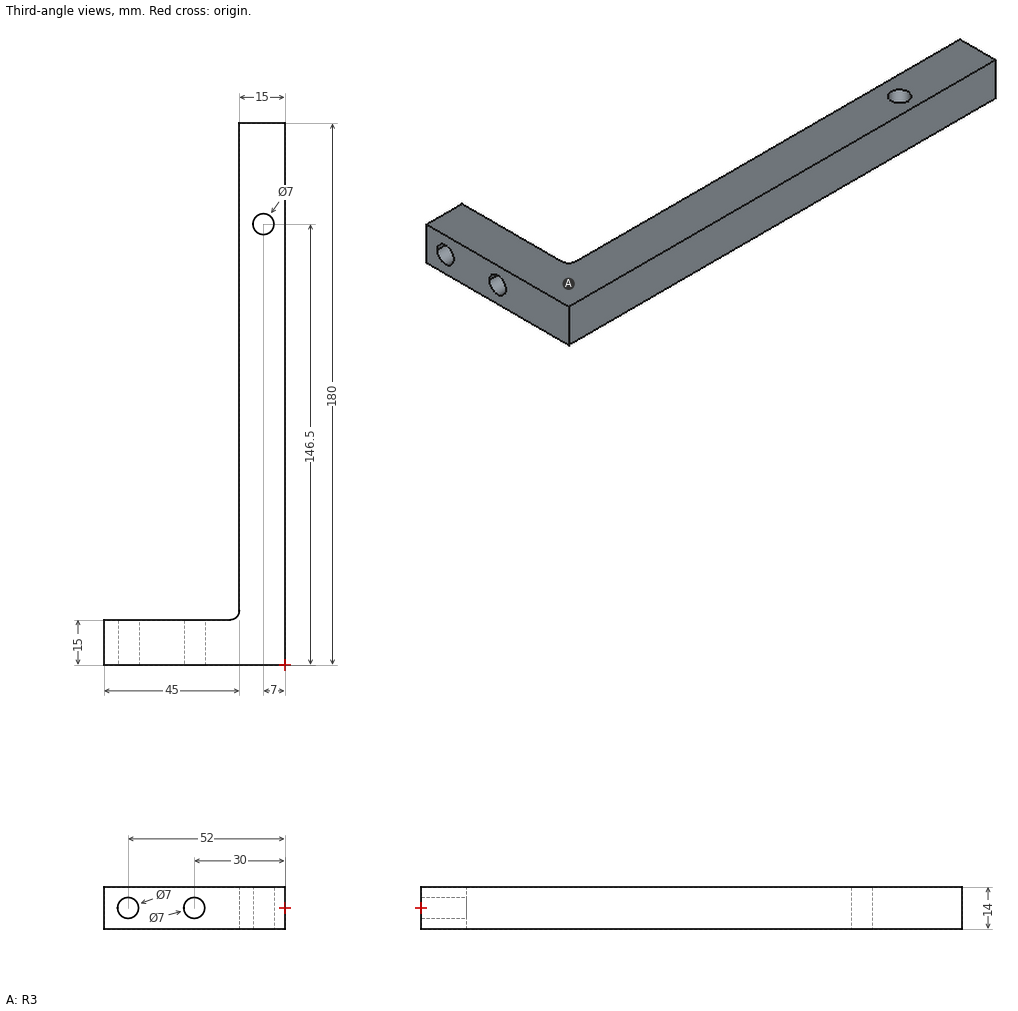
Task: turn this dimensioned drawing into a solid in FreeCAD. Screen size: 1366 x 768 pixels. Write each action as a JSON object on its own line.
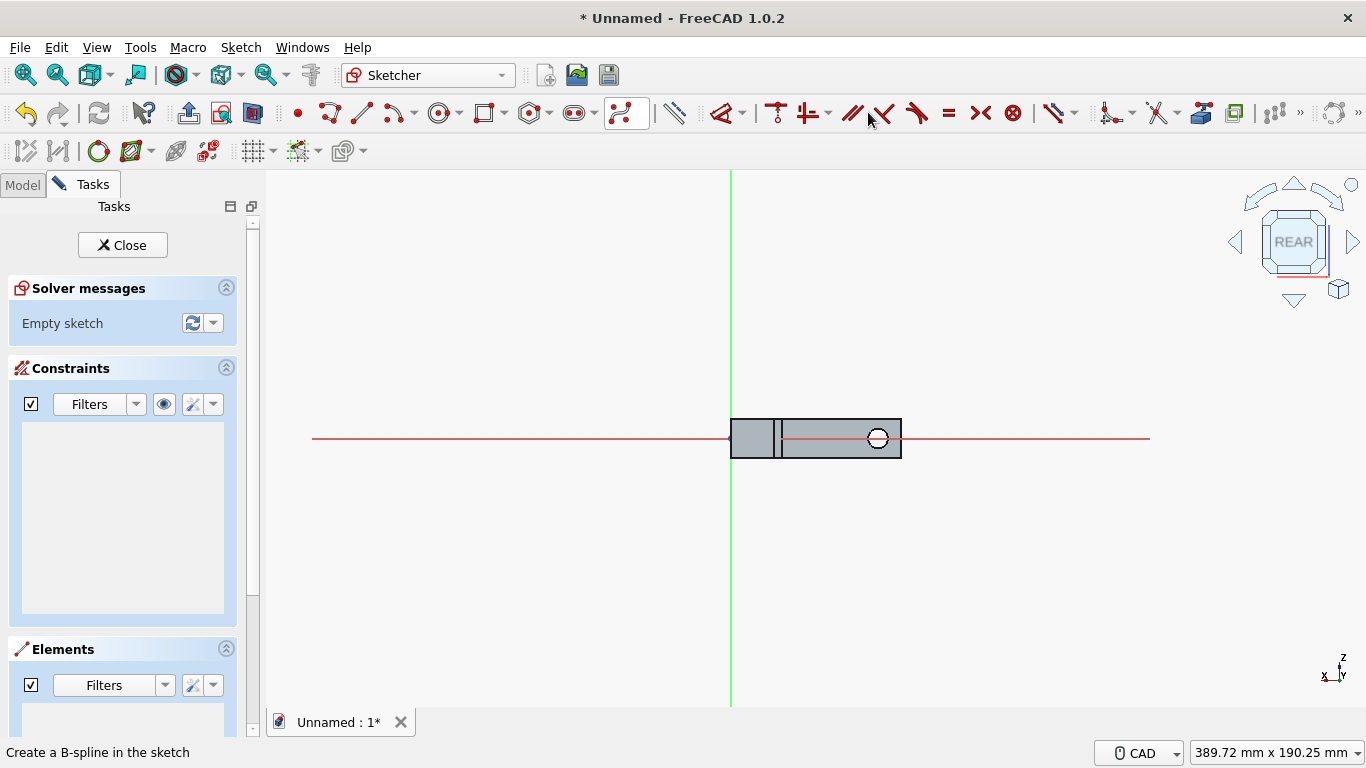
{"action": "left_click", "coordinate": [254, 114]}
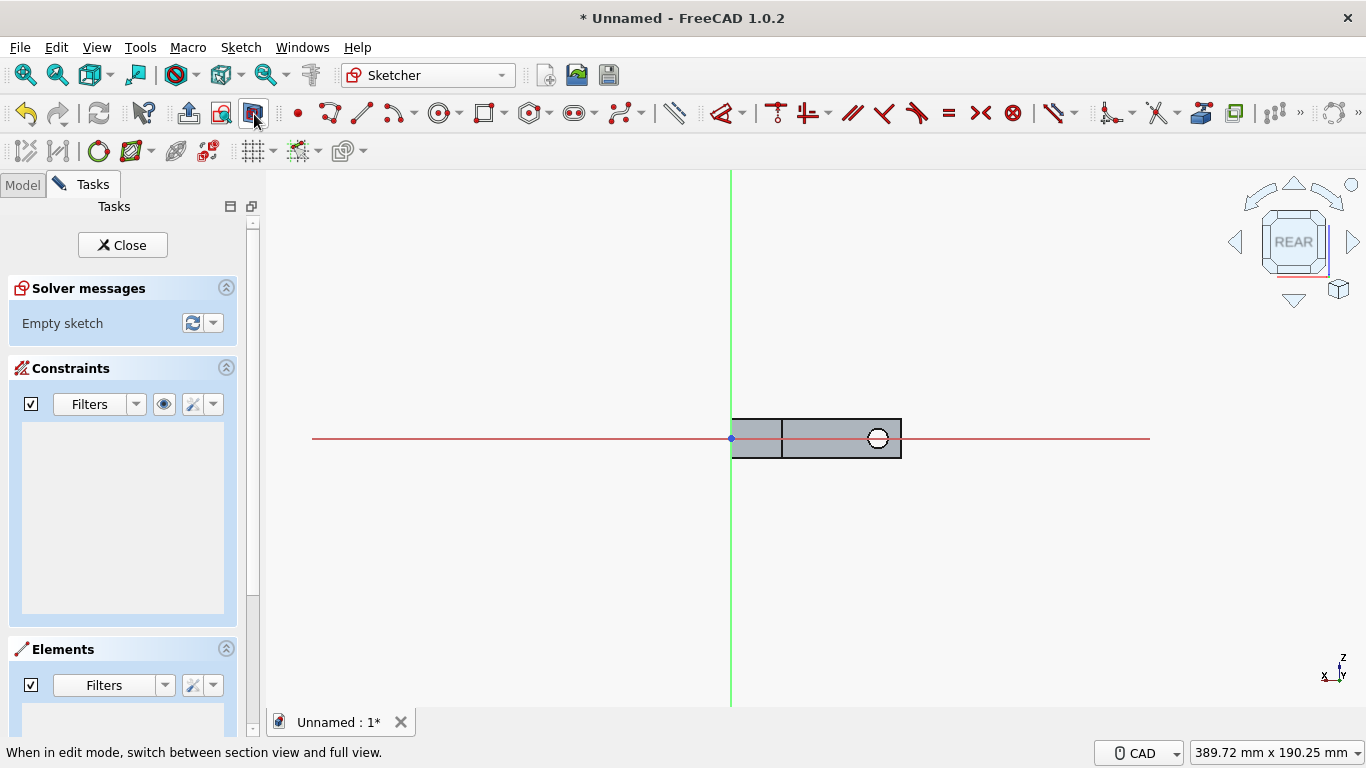
{"action": "scroll", "coordinate": [820, 439], "scroll_direction": "up", "scroll_amount": 14}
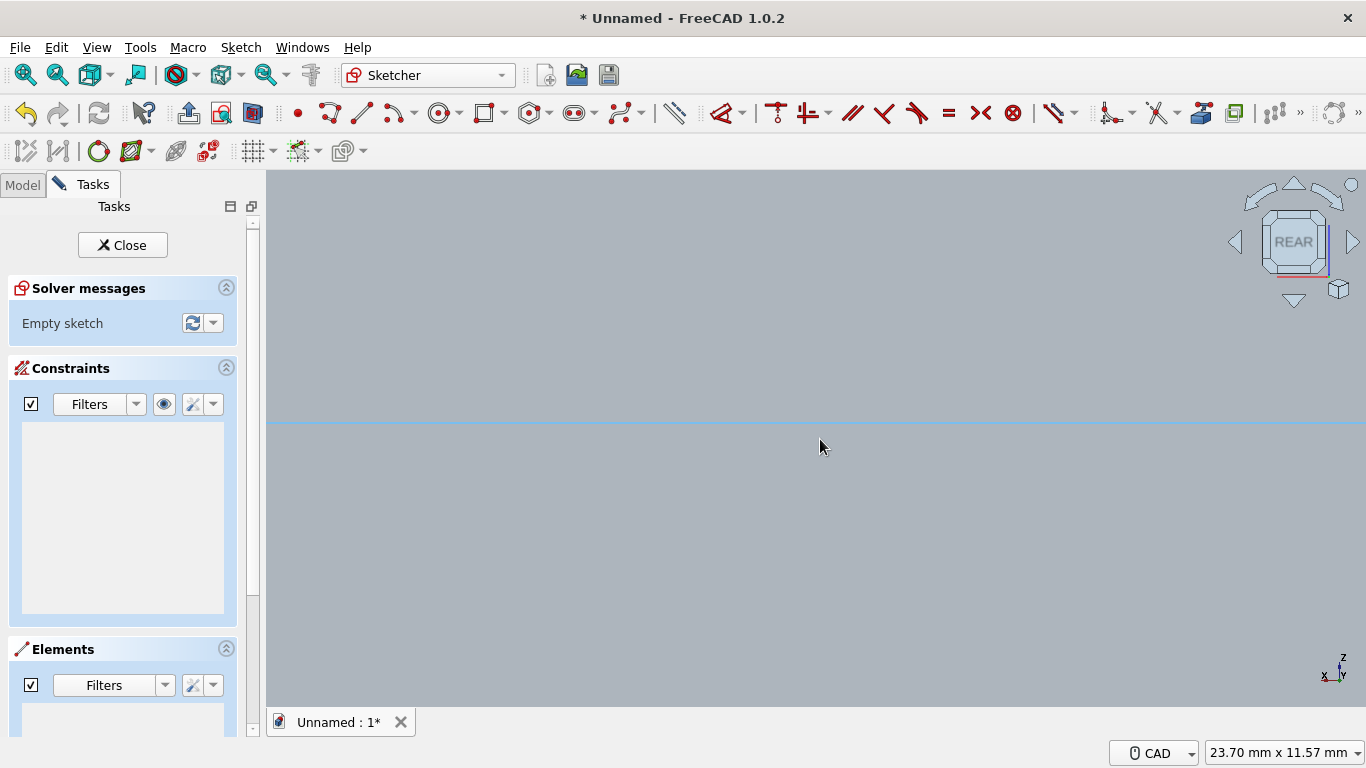
{"action": "left_click", "coordinate": [440, 114]}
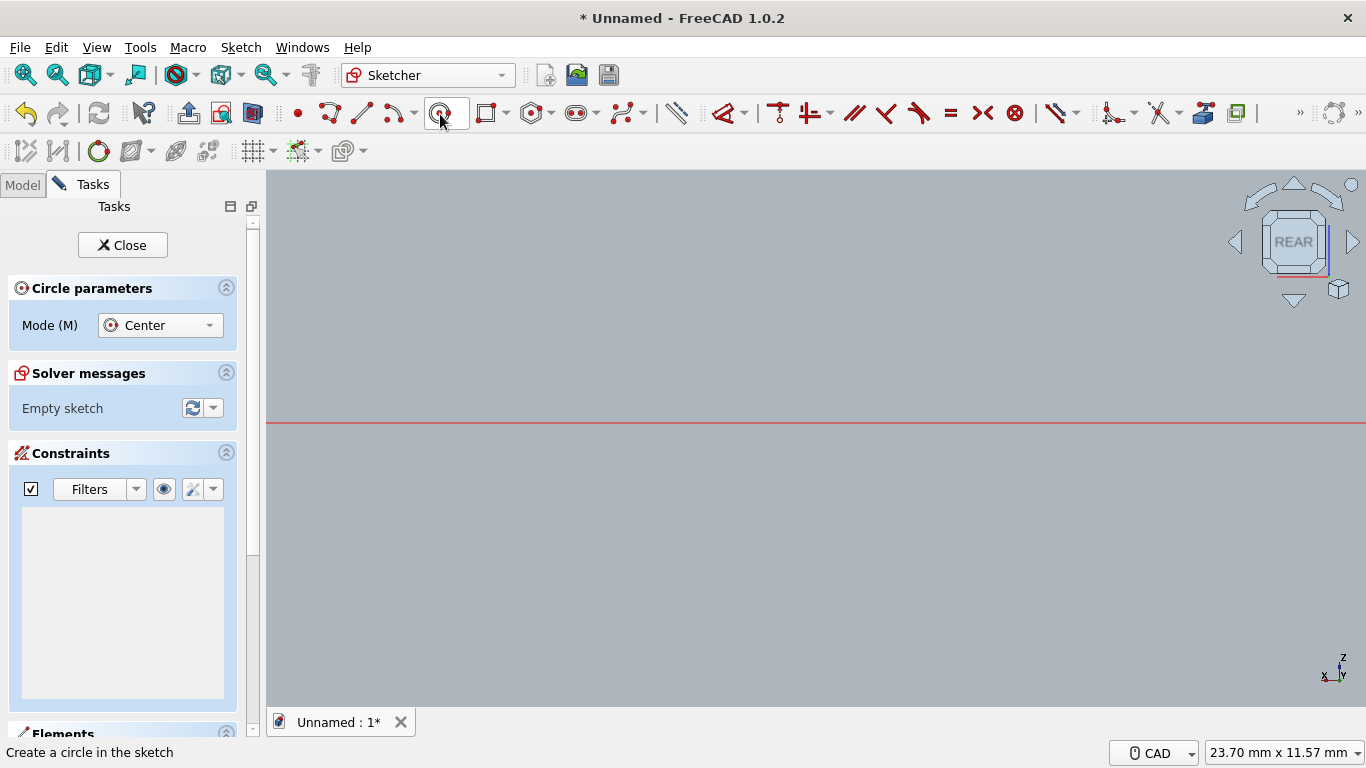
{"action": "left_click", "coordinate": [746, 423]}
{"action": "mouse_move", "coordinate": [861, 308]}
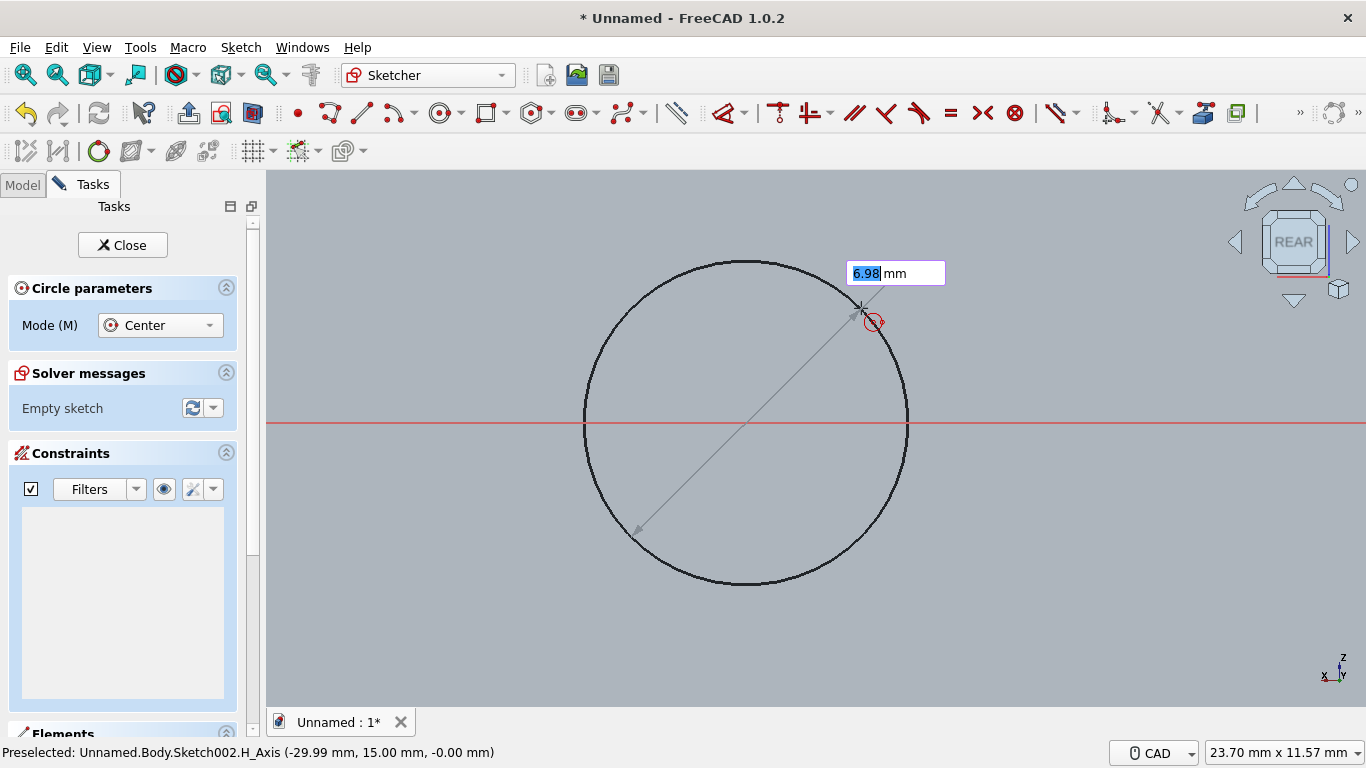
{"action": "type", "text": "7"}
{"action": "key", "text": "Return"}
{"action": "key", "text": "Escape"}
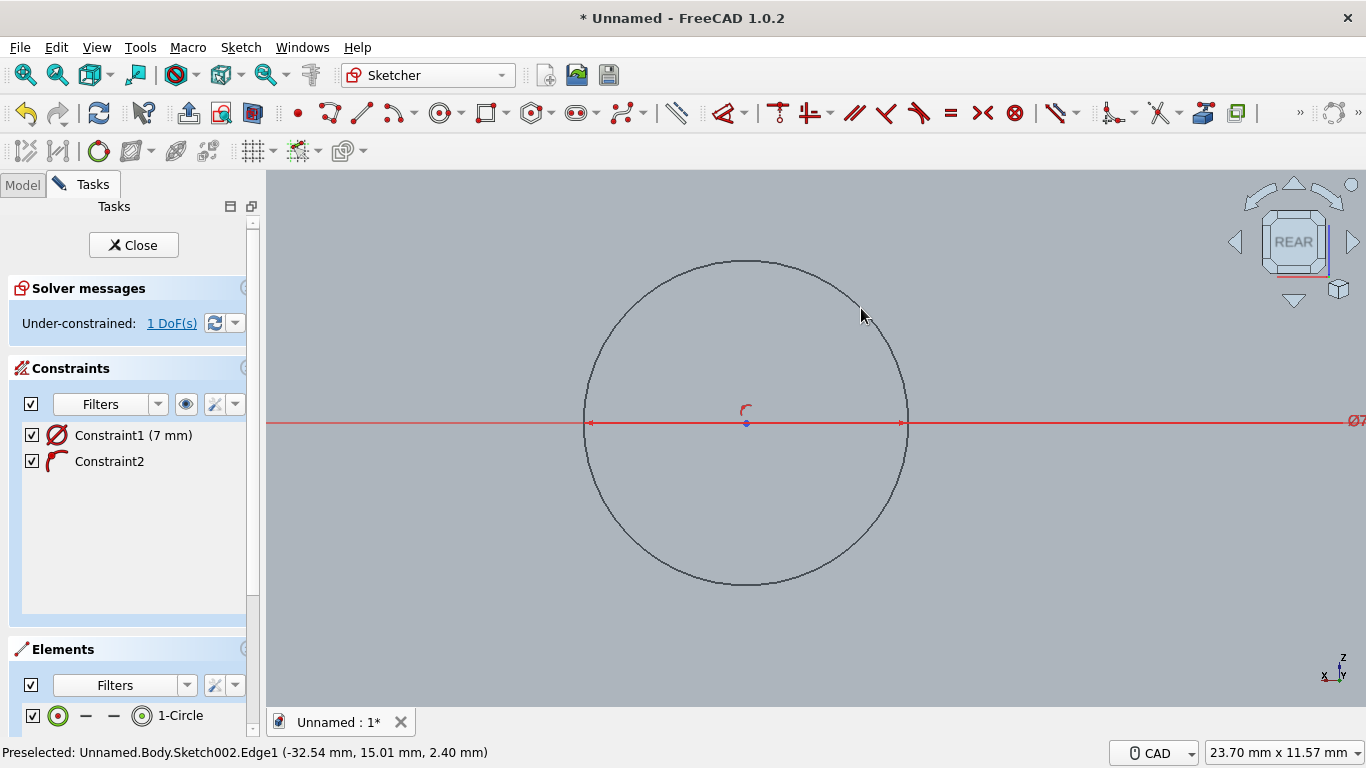
{"action": "left_click", "coordinate": [724, 114]}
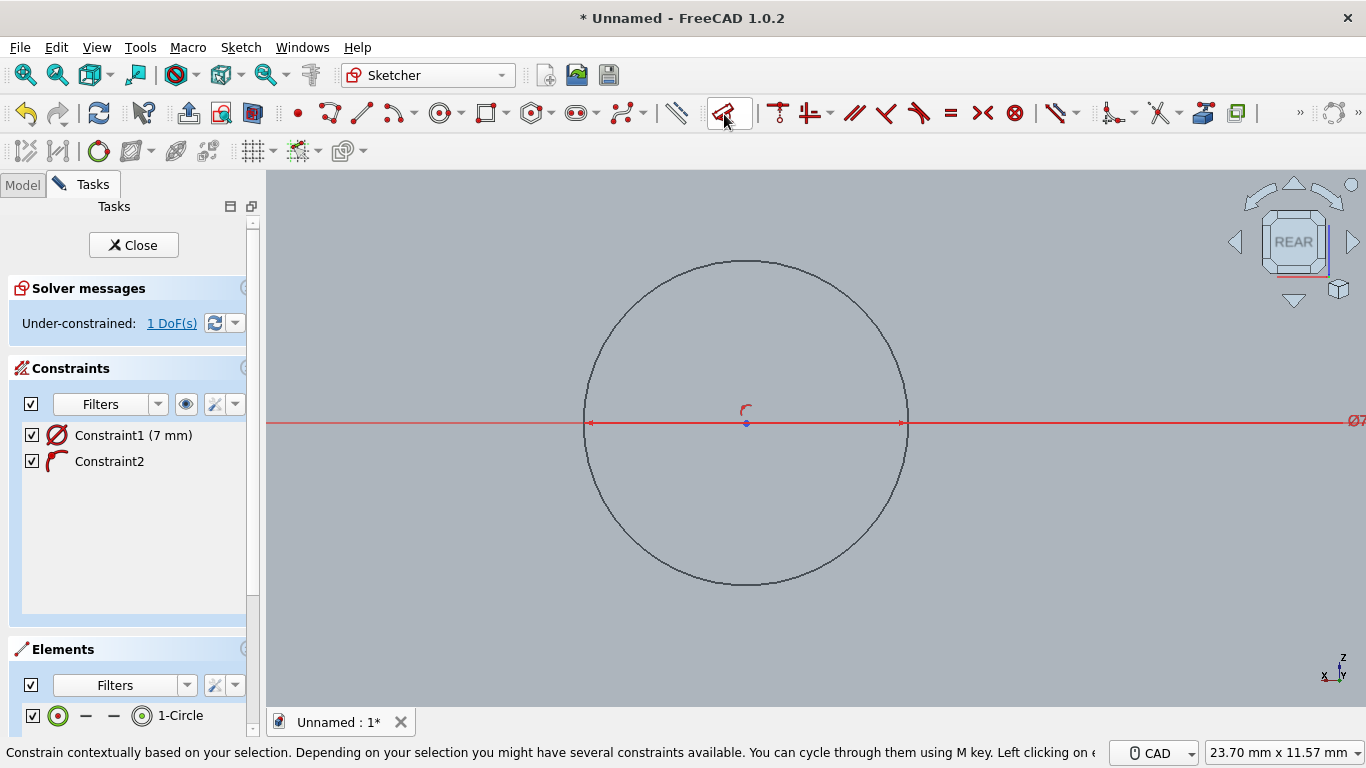
{"action": "left_click", "coordinate": [746, 423]}
{"action": "left_click", "coordinate": [520, 457]}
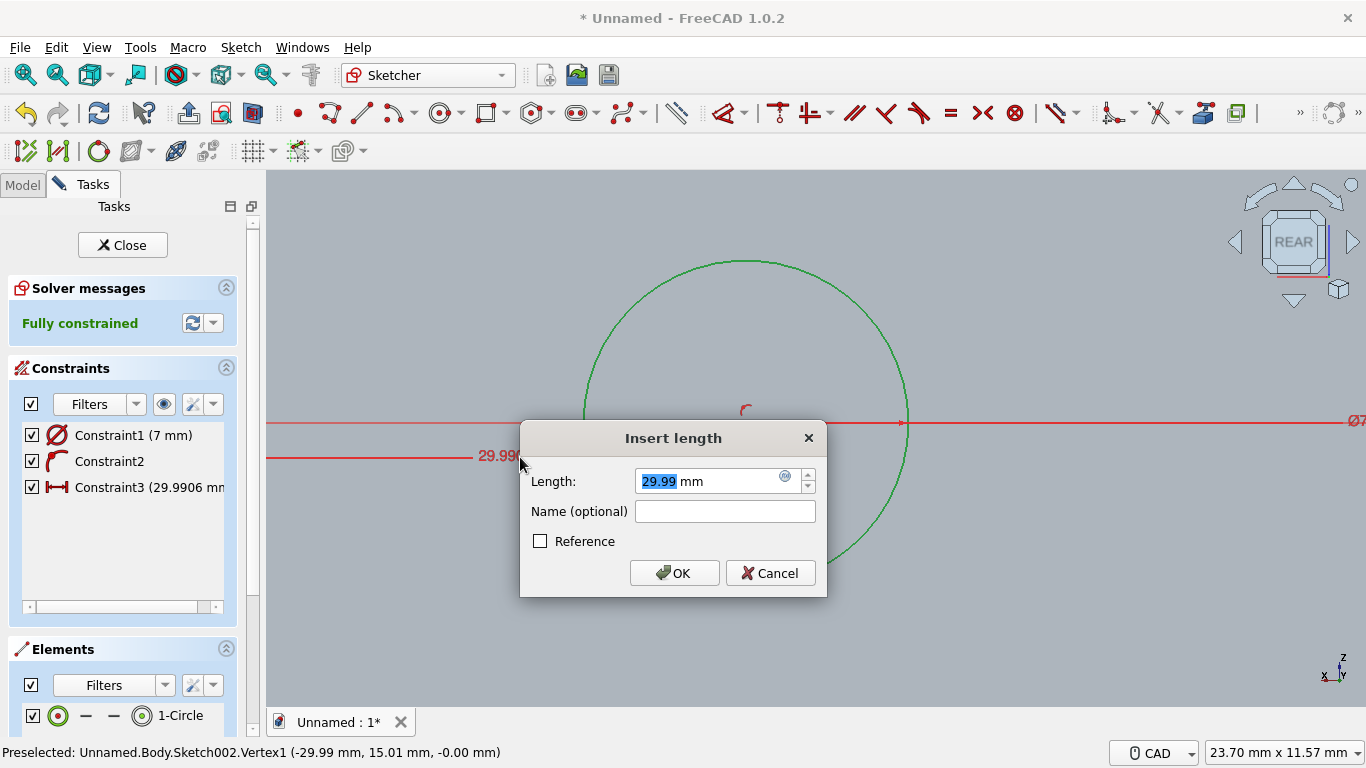
{"action": "type", "text": "30"}
{"action": "key", "text": "Return"}
{"action": "key", "text": "Escape"}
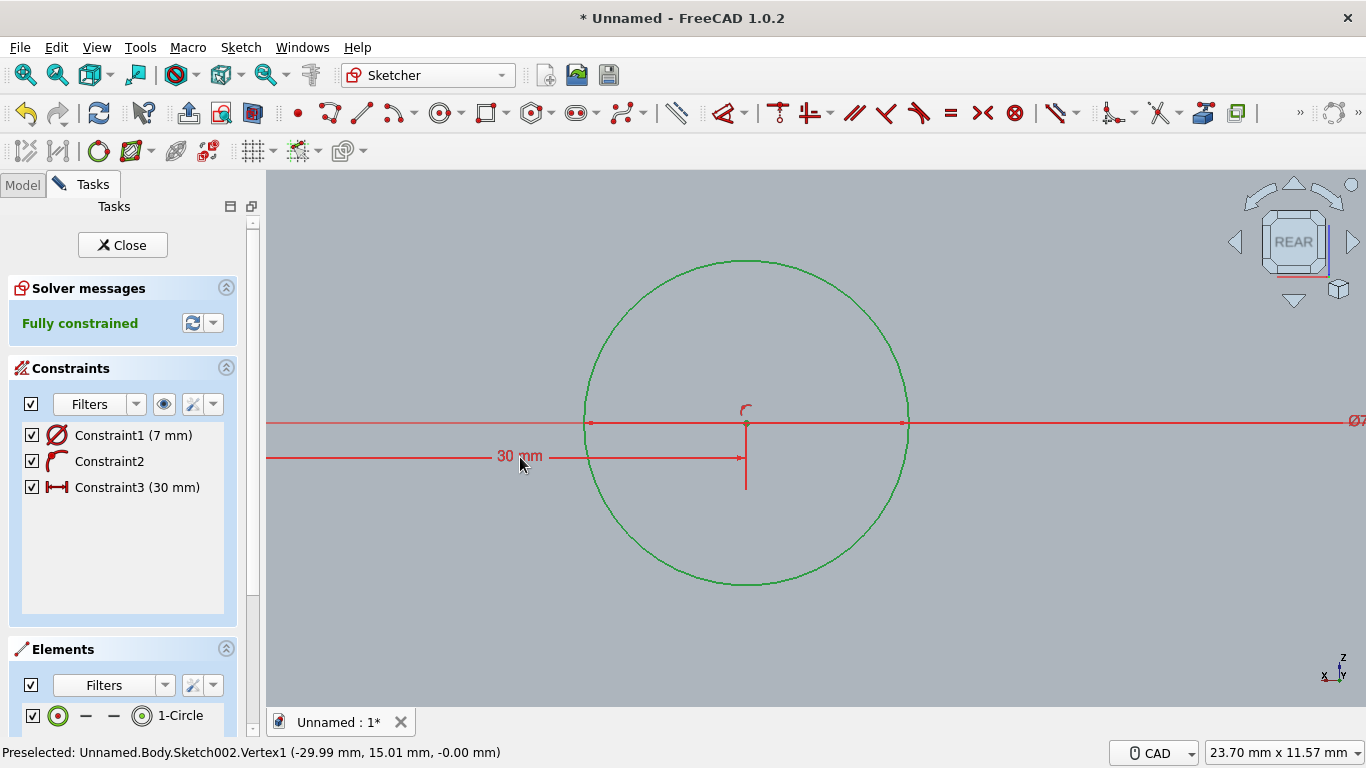
{"action": "left_click", "coordinate": [123, 245]}